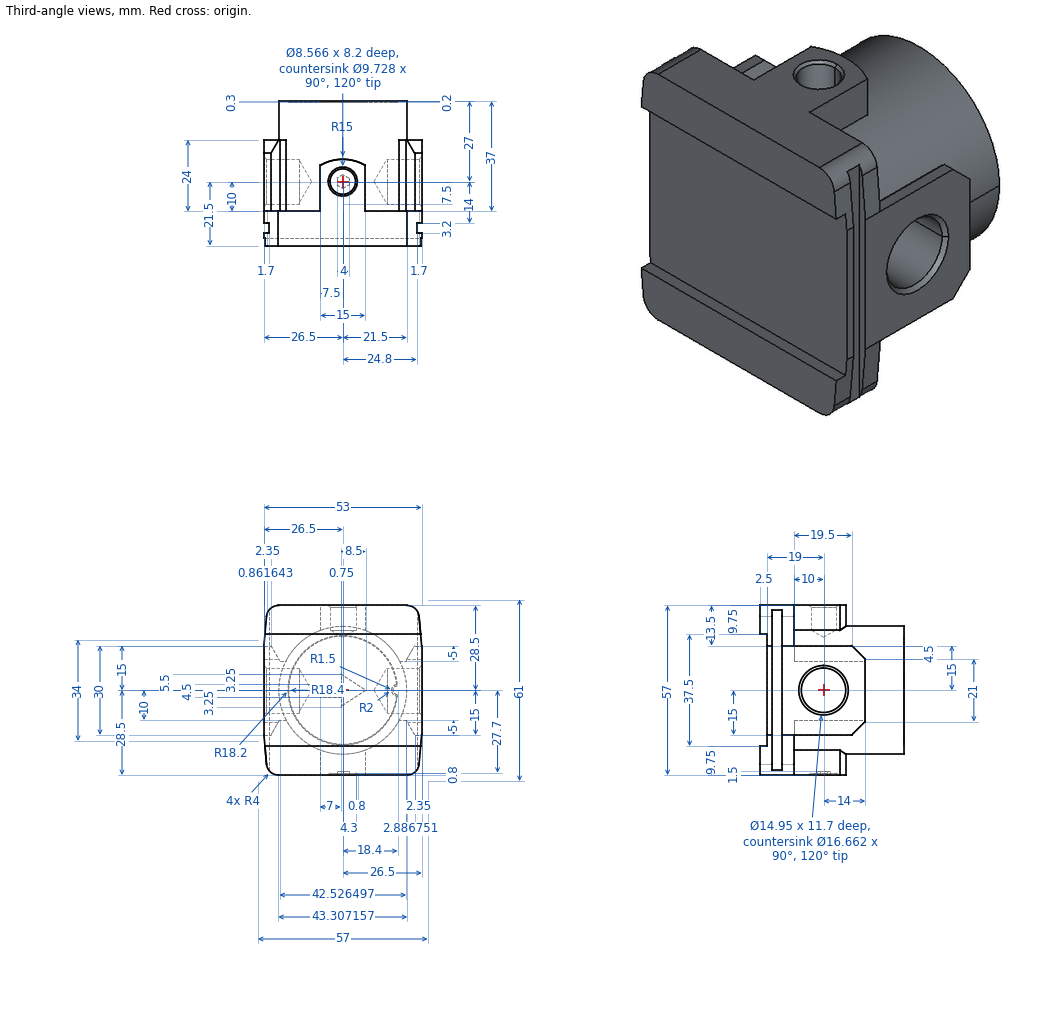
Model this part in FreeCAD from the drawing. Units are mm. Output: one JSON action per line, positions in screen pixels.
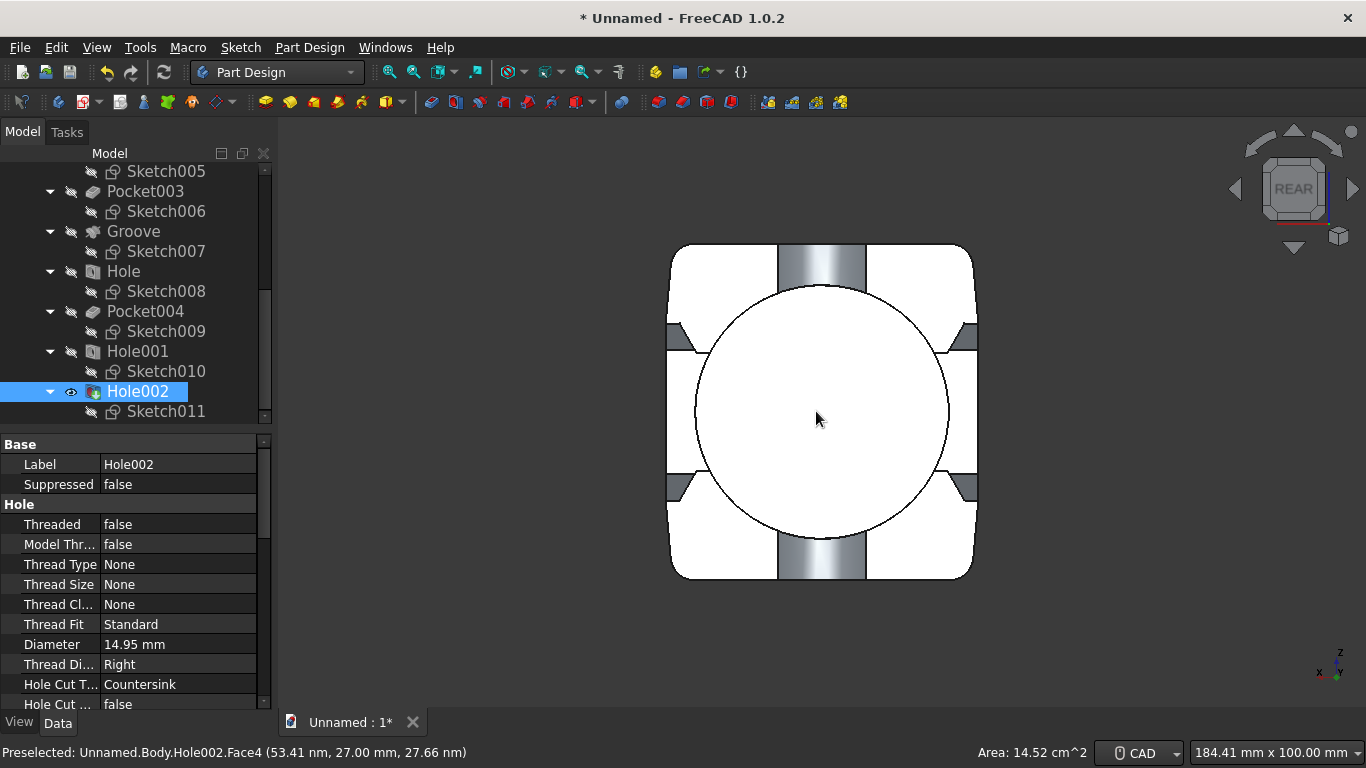
{"action": "left_click", "coordinate": [84, 102]}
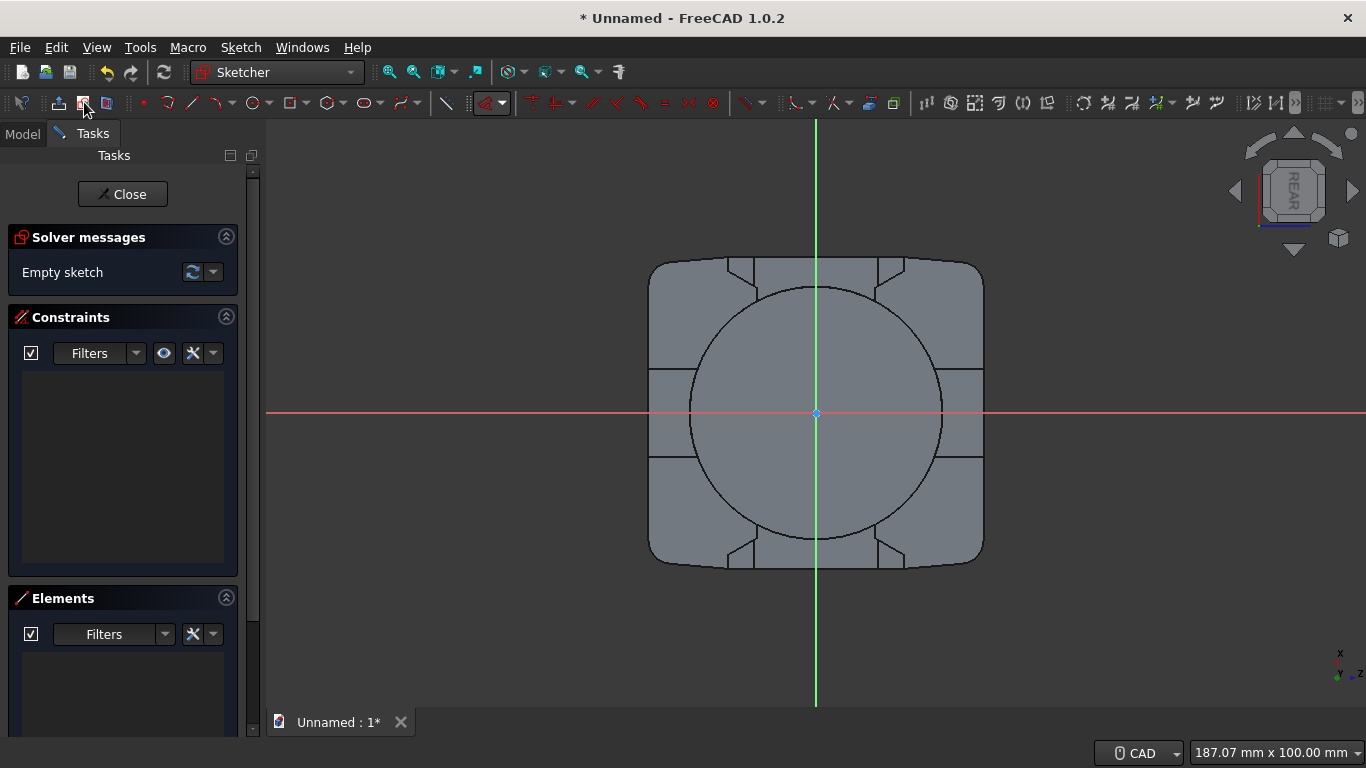
{"action": "scroll", "coordinate": [838, 413], "scroll_direction": "up", "scroll_amount": 7}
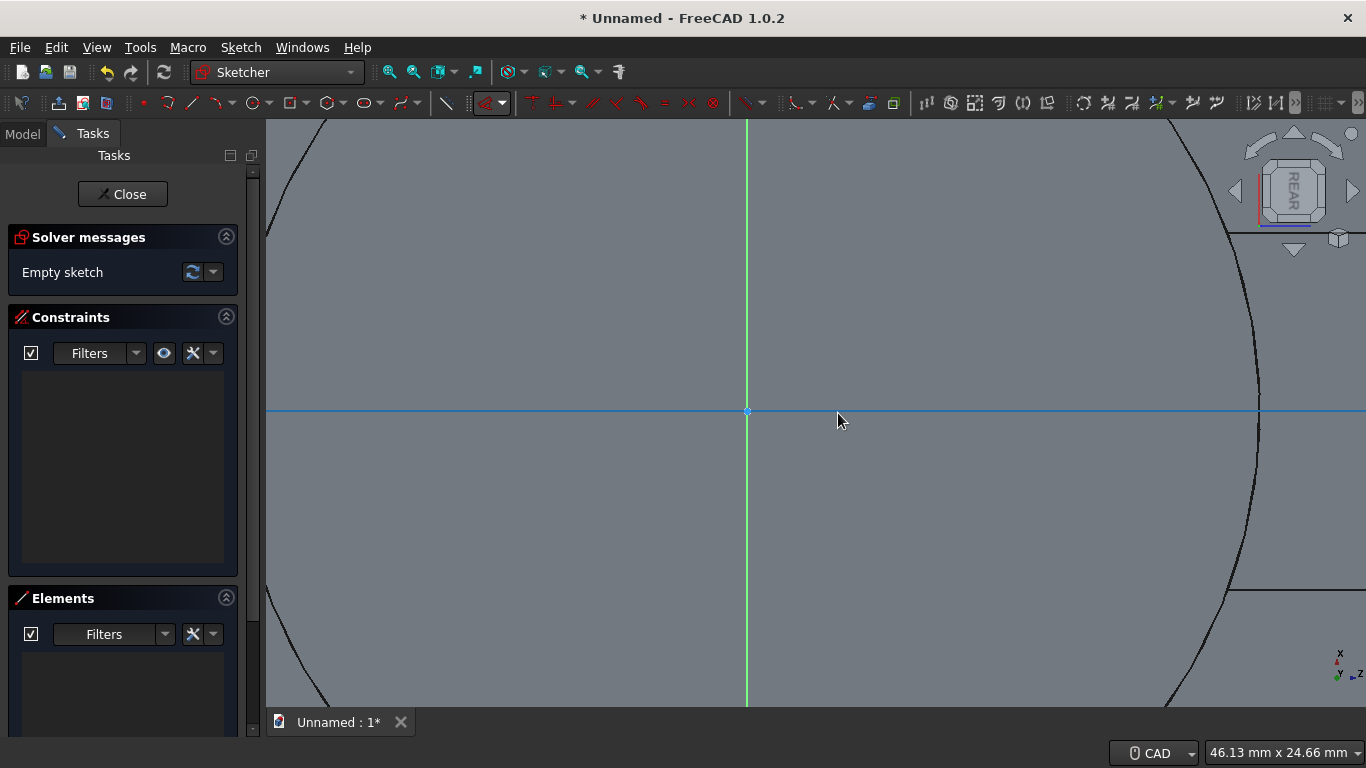
{"action": "left_click", "coordinate": [168, 104]}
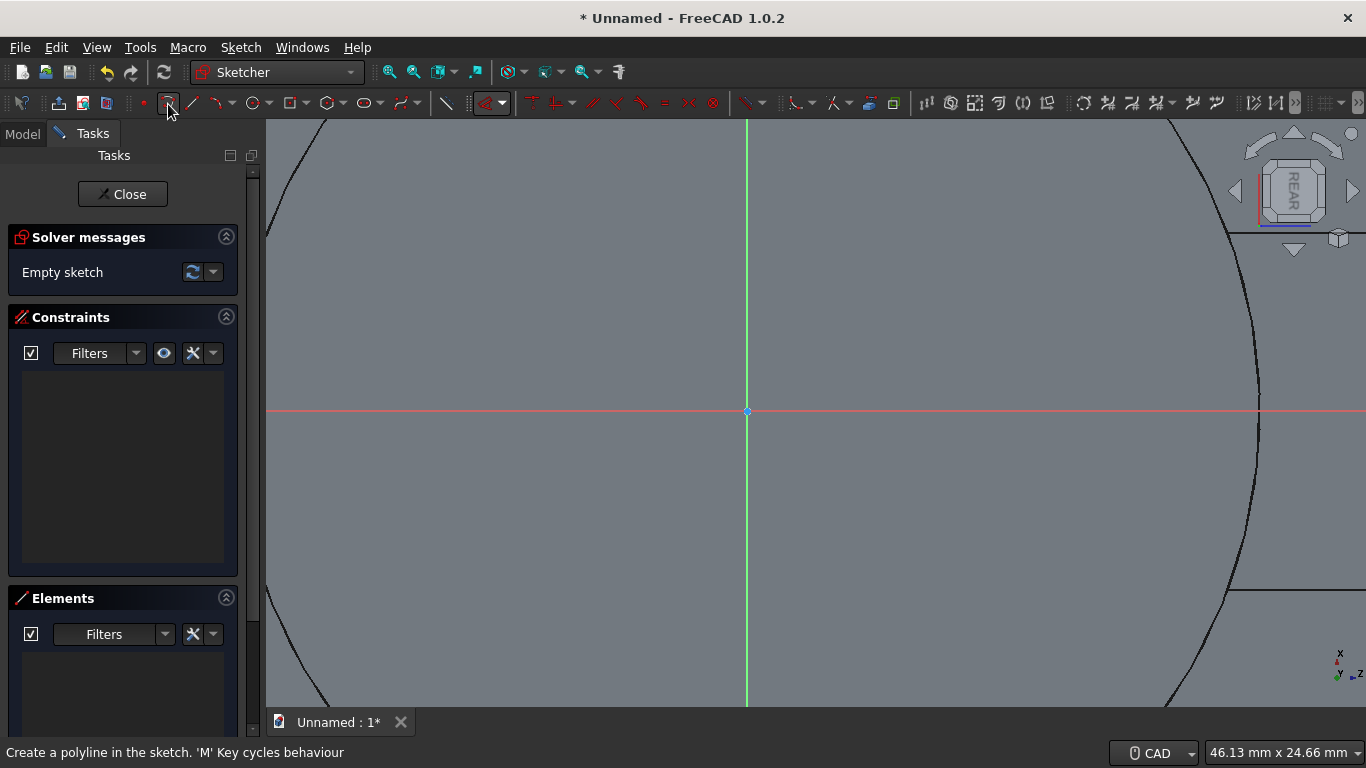
{"action": "left_click", "coordinate": [801, 429]}
{"action": "left_click", "coordinate": [878, 429]}
{"action": "left_click", "coordinate": [747, 227]}
{"action": "left_click", "coordinate": [616, 429]}
{"action": "left_click", "coordinate": [694, 429]}
{"action": "left_click", "coordinate": [694, 596]}
{"action": "left_click", "coordinate": [801, 596]}
{"action": "left_click", "coordinate": [801, 430]}
{"action": "key", "text": "Escape"}
{"action": "key", "text": "Escape"}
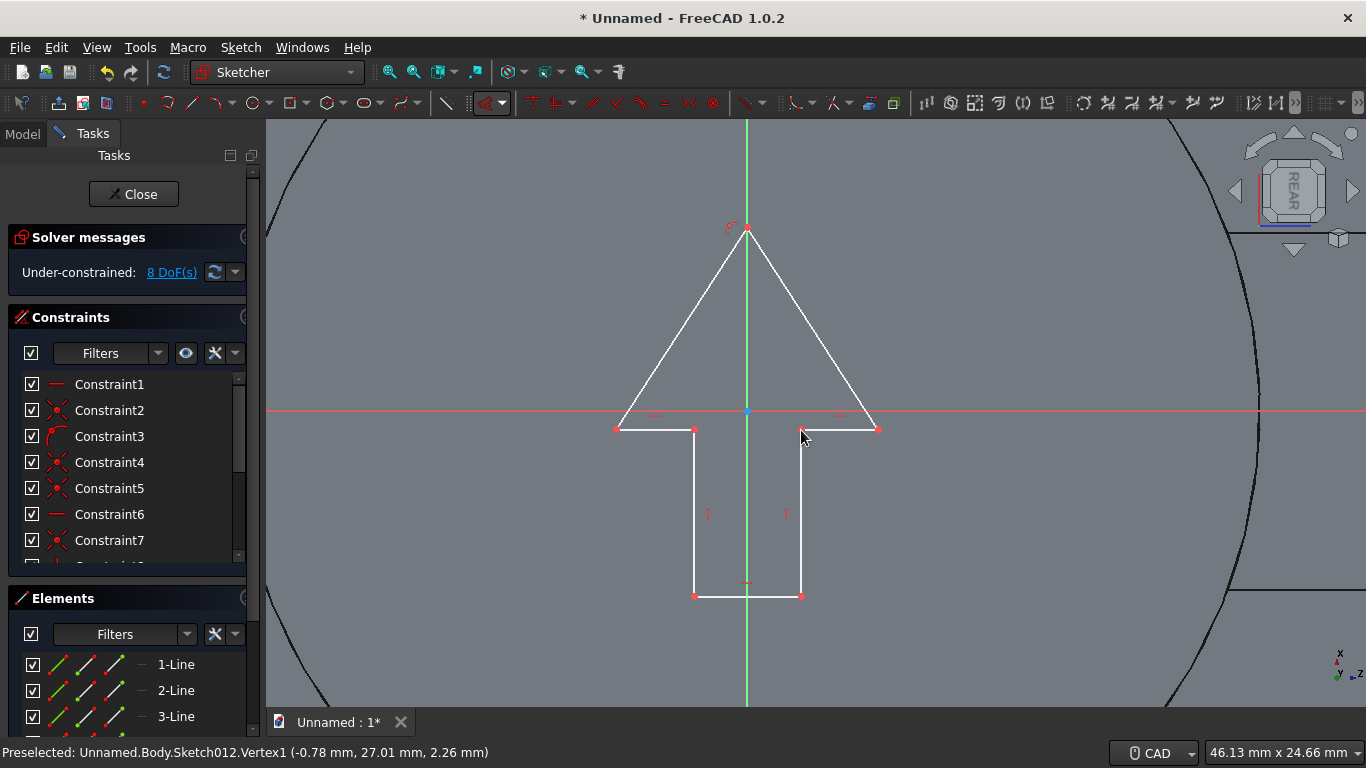
{"action": "left_click", "coordinate": [694, 480]}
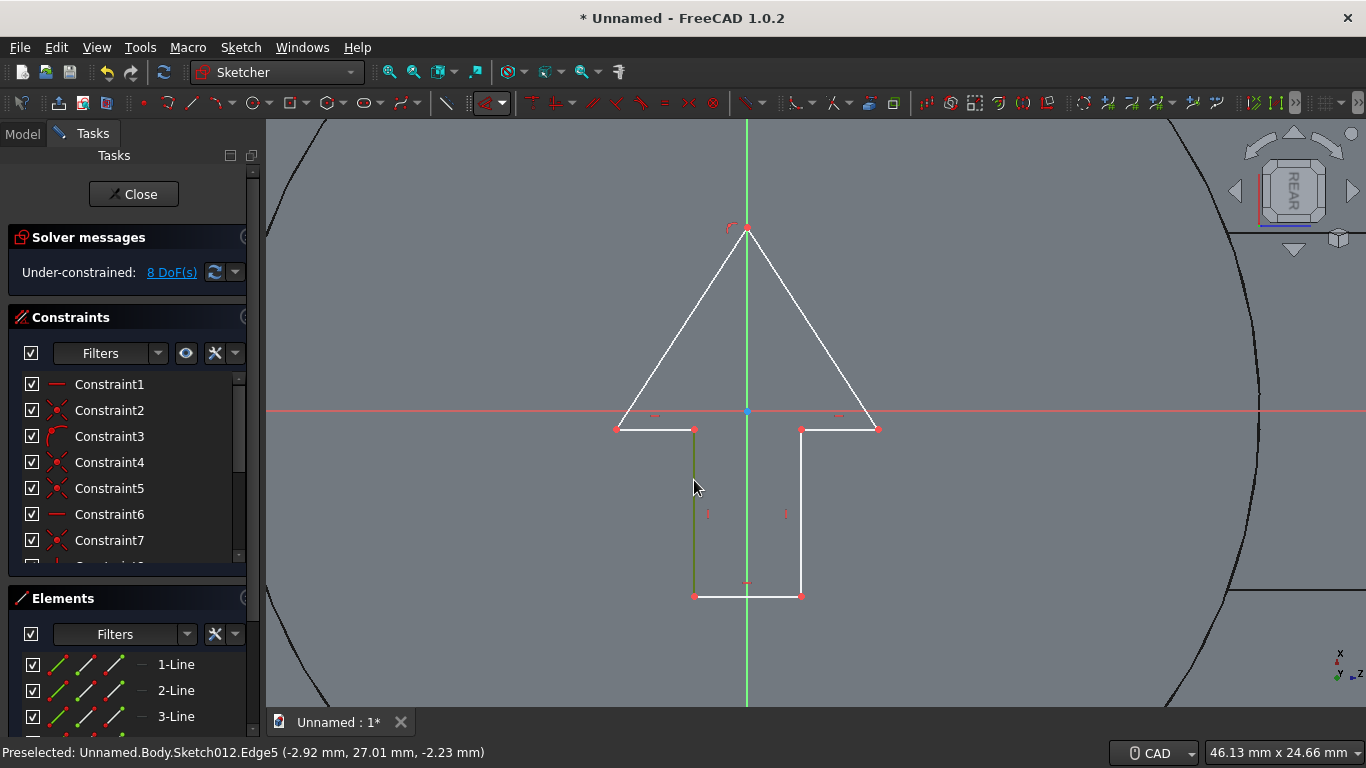
{"action": "key", "text": "i"}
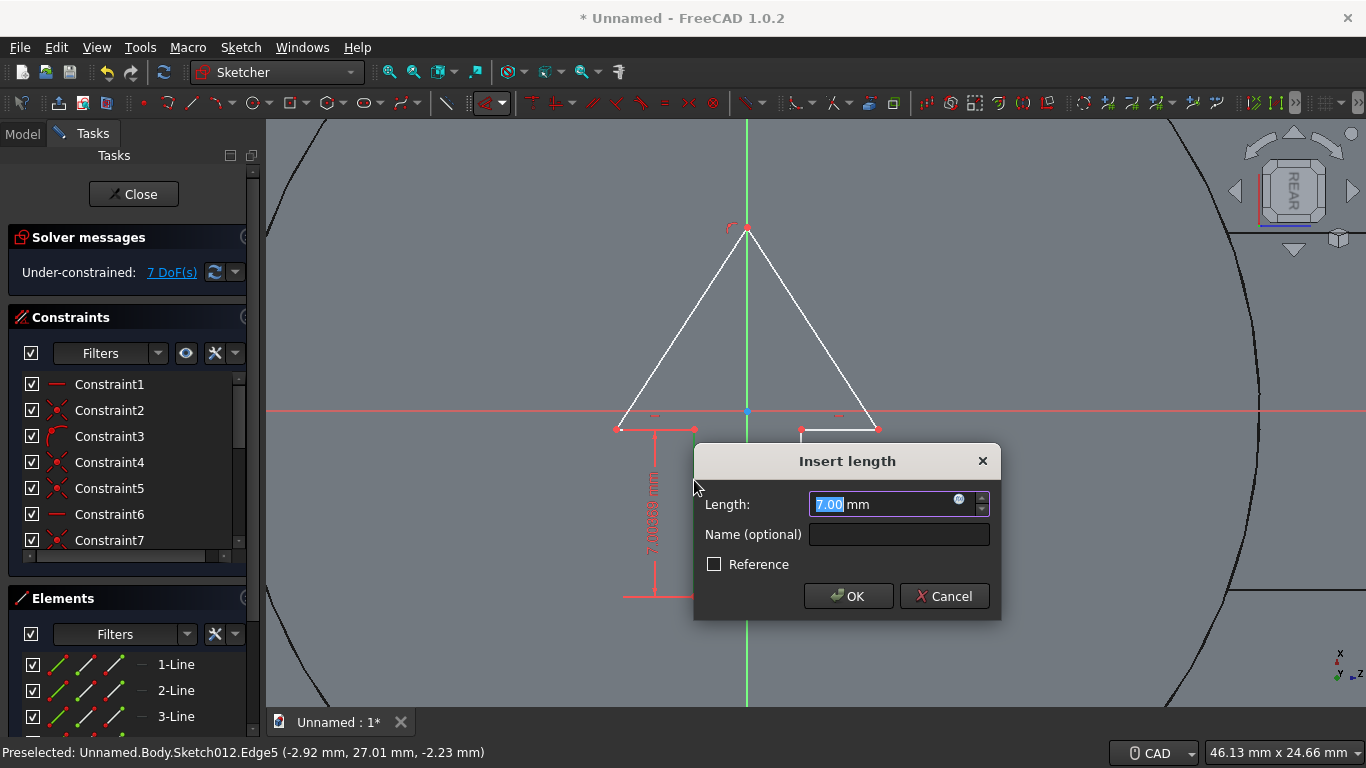
{"action": "type", "text": "7"}
{"action": "key", "text": "Return"}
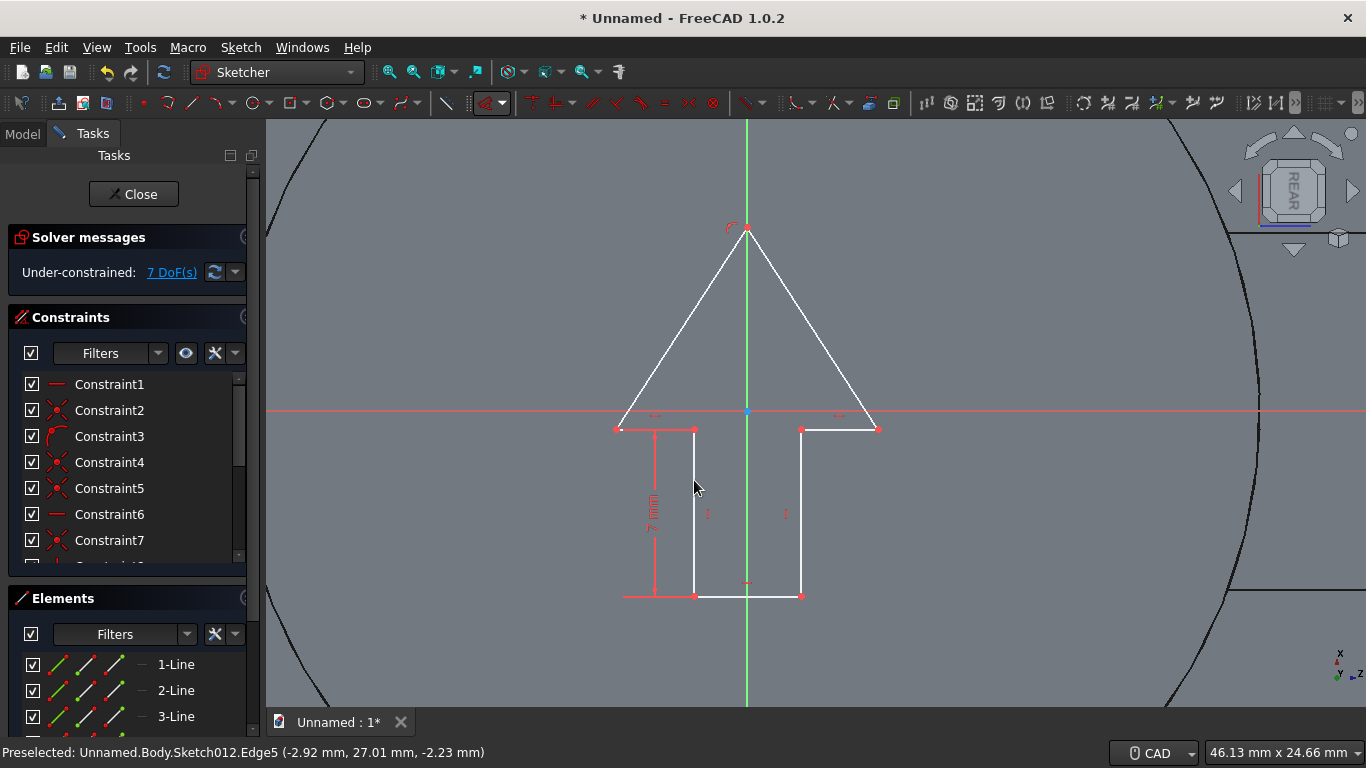
{"action": "left_click", "coordinate": [801, 547]}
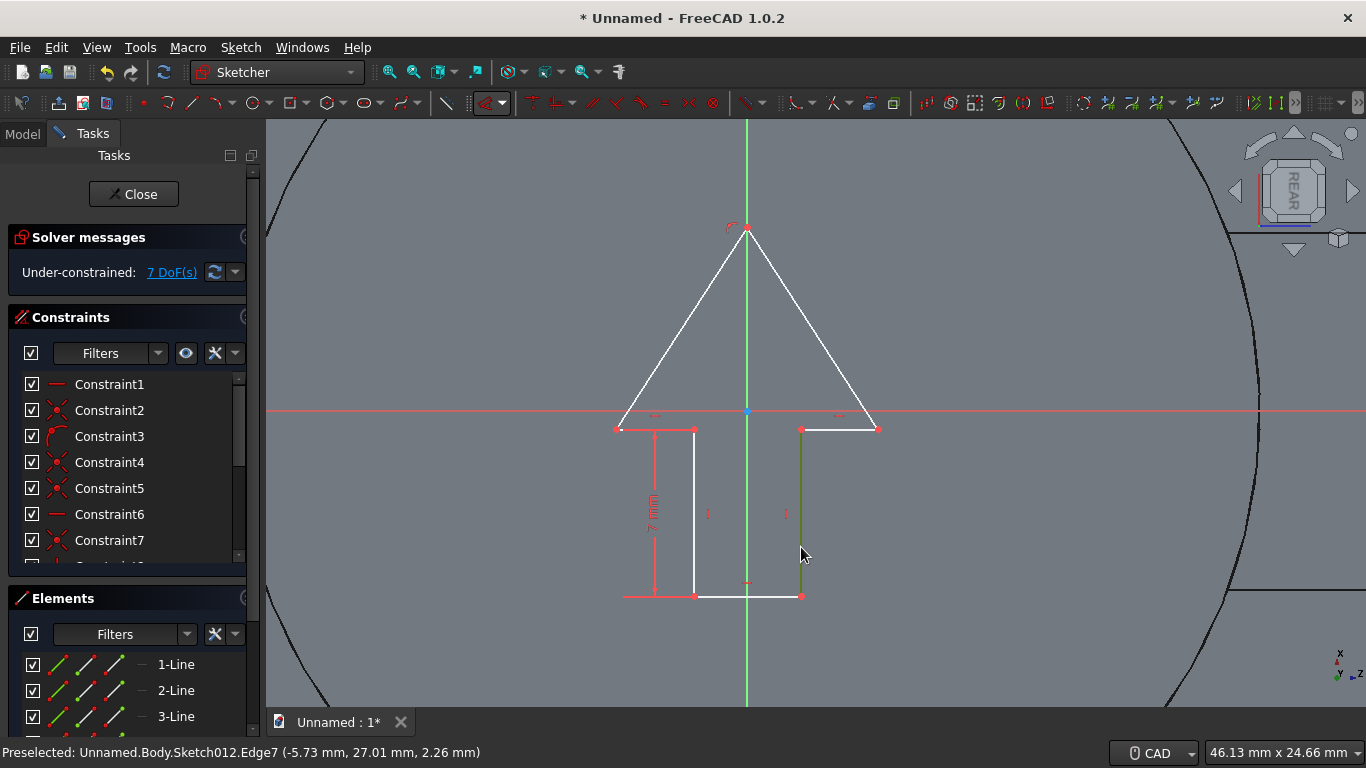
{"action": "key", "text": "i"}